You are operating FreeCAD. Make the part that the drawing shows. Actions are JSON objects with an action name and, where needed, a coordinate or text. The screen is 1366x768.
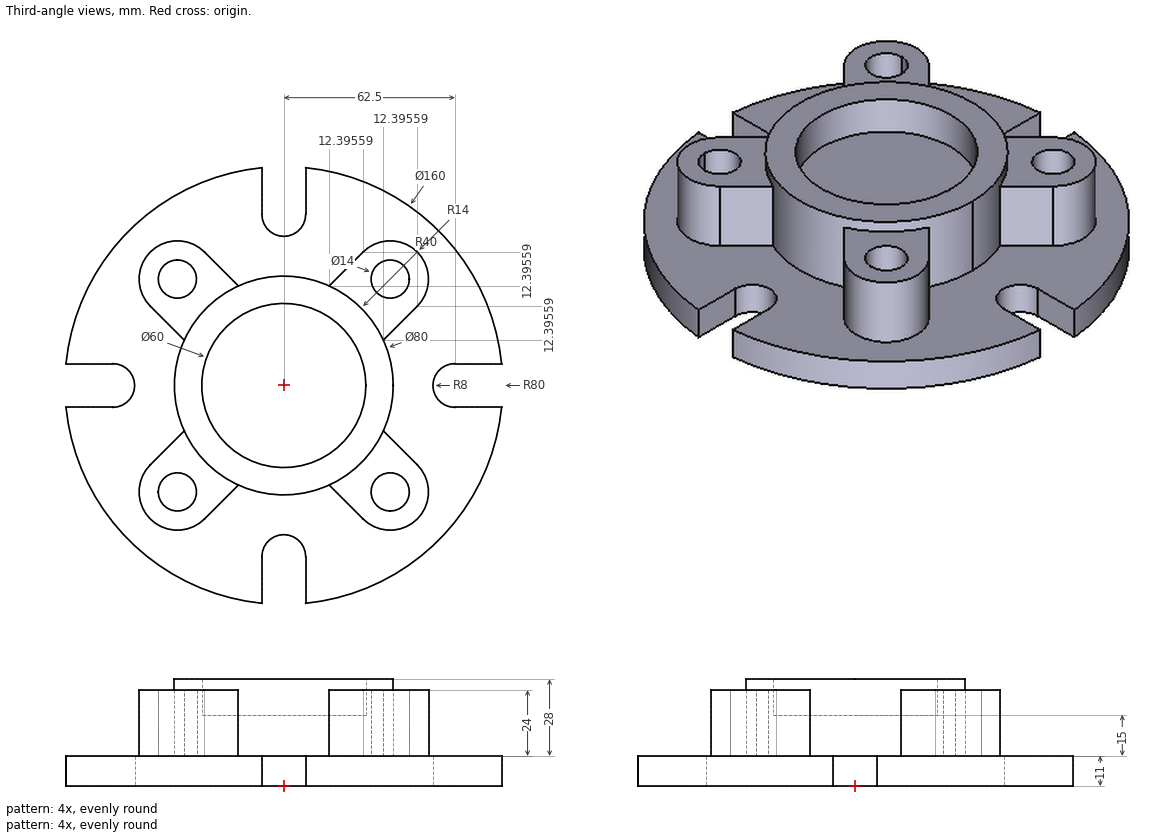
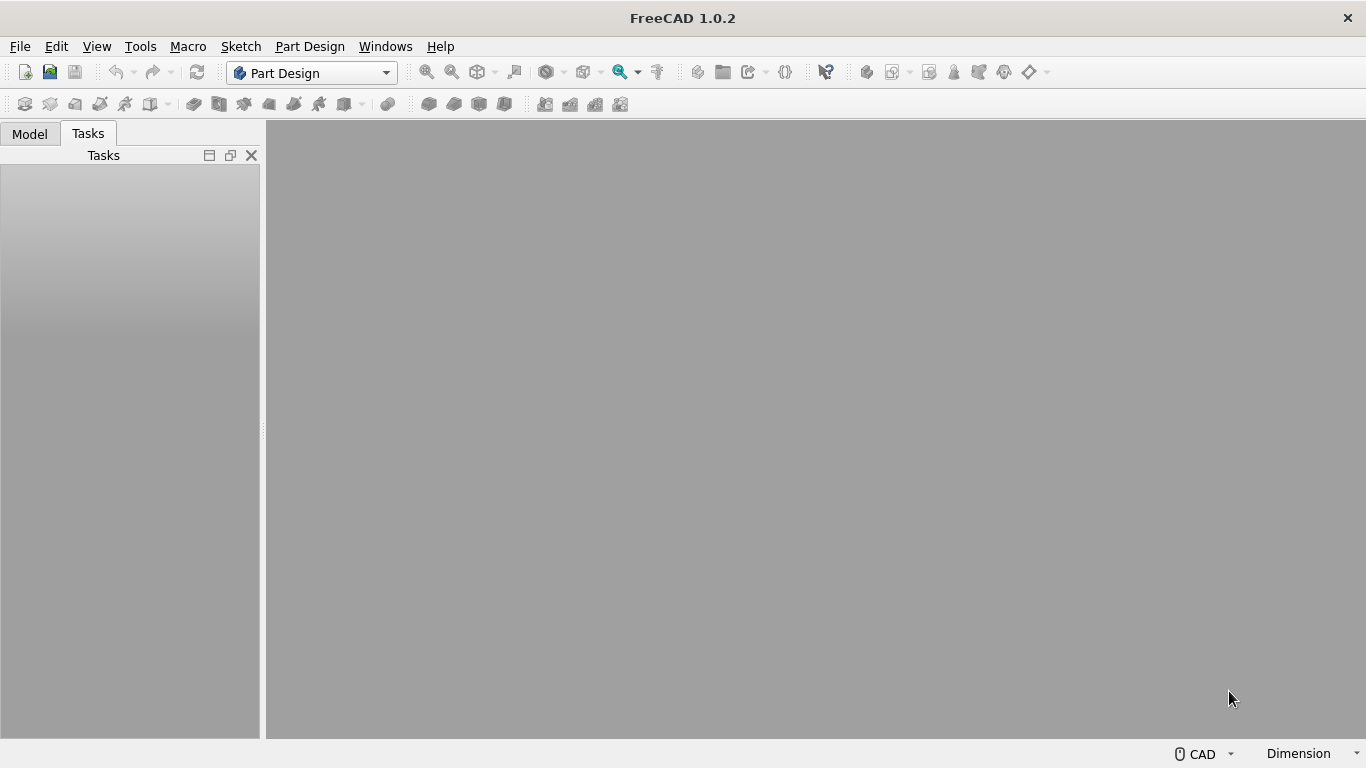
{"action": "left_click", "coordinate": [25, 72]}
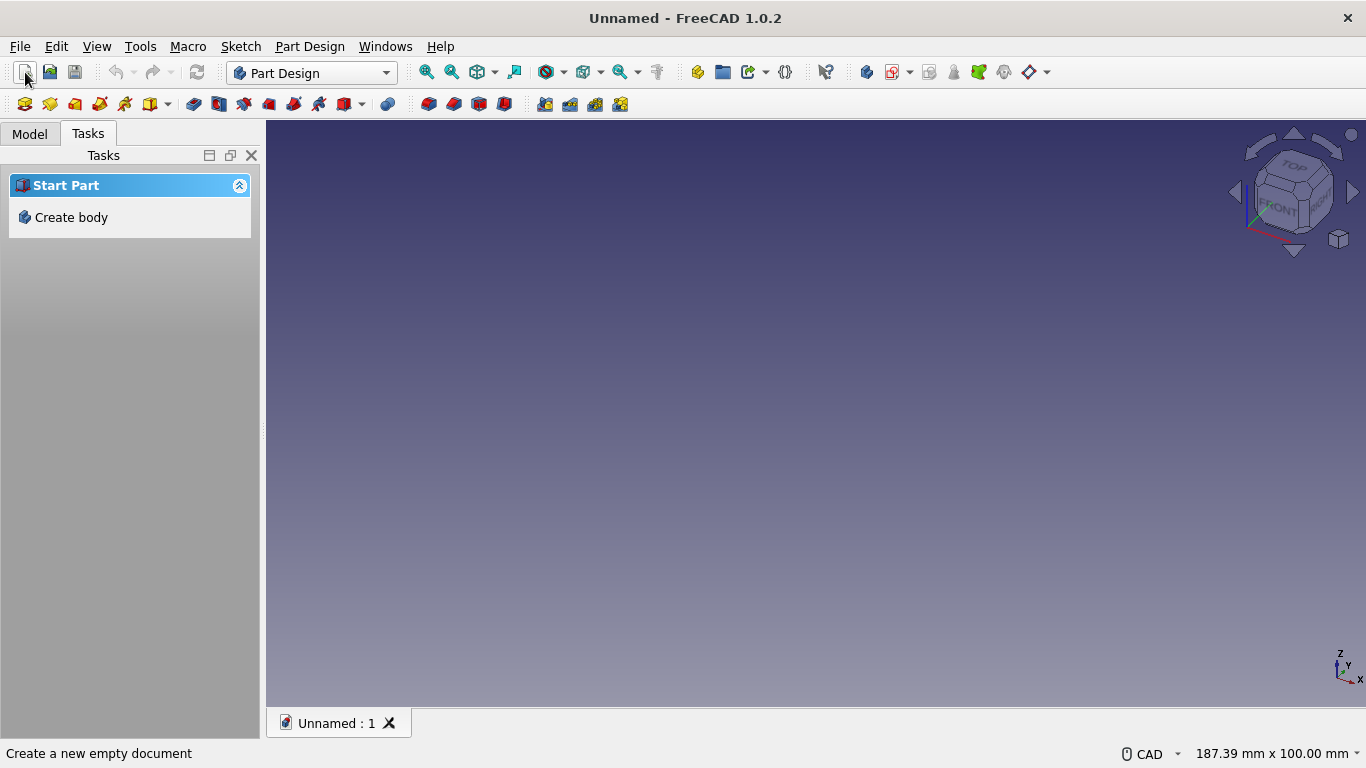
{"action": "left_click", "coordinate": [892, 72]}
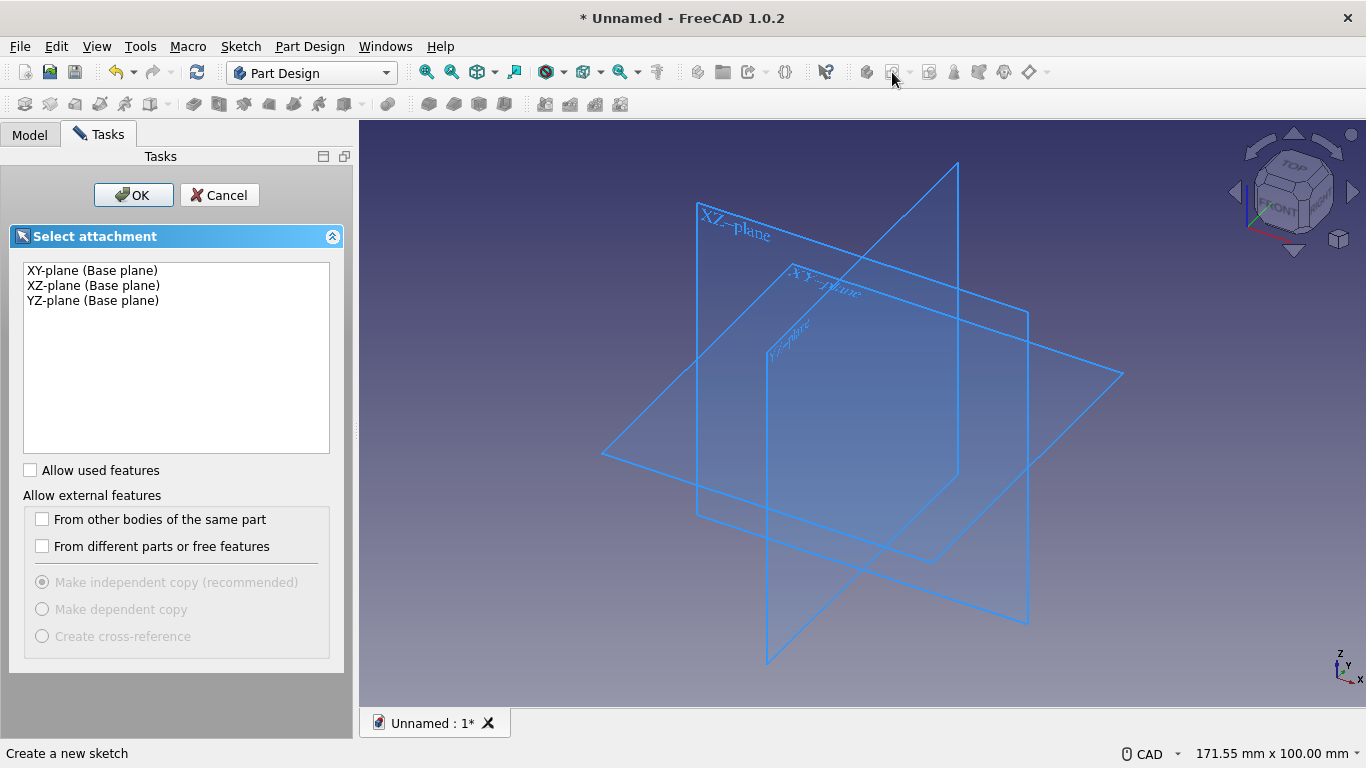
{"action": "left_click", "coordinate": [84, 270]}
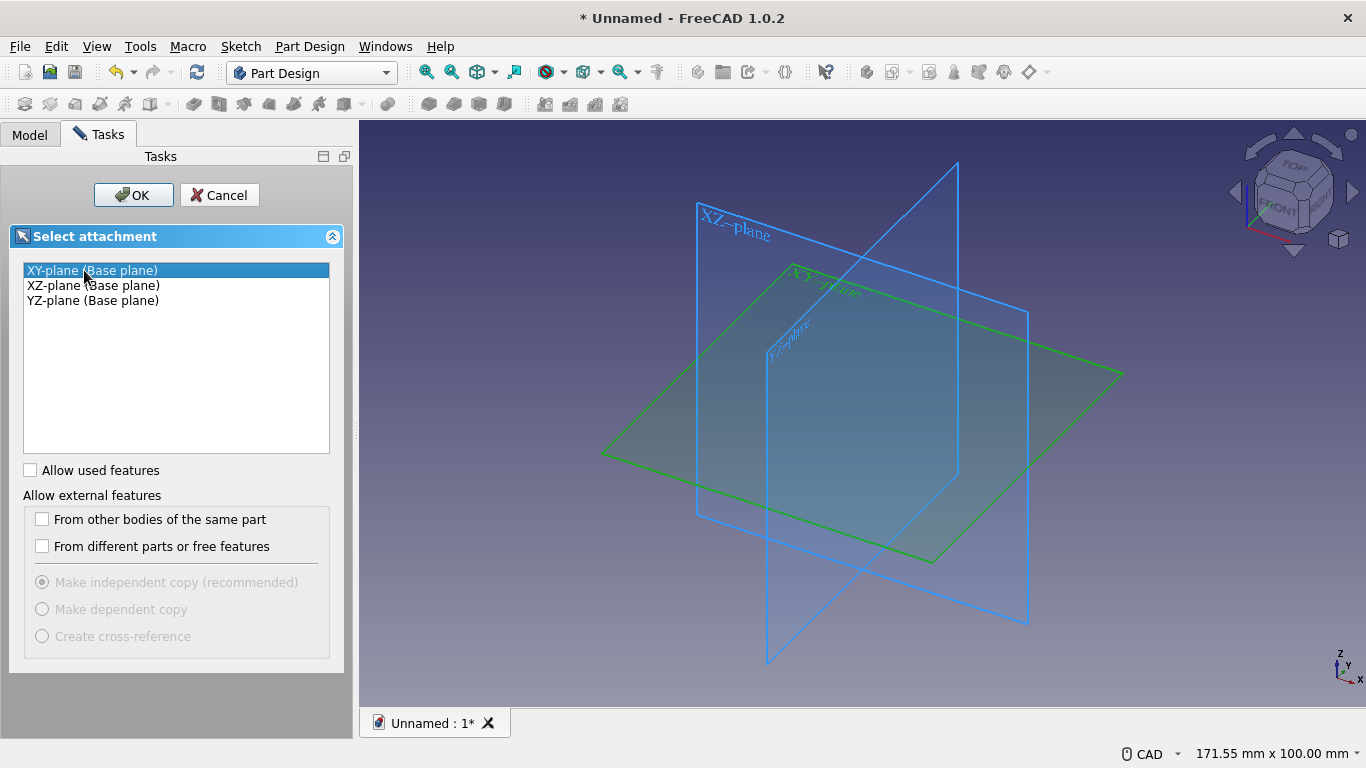
{"action": "left_click", "coordinate": [134, 195]}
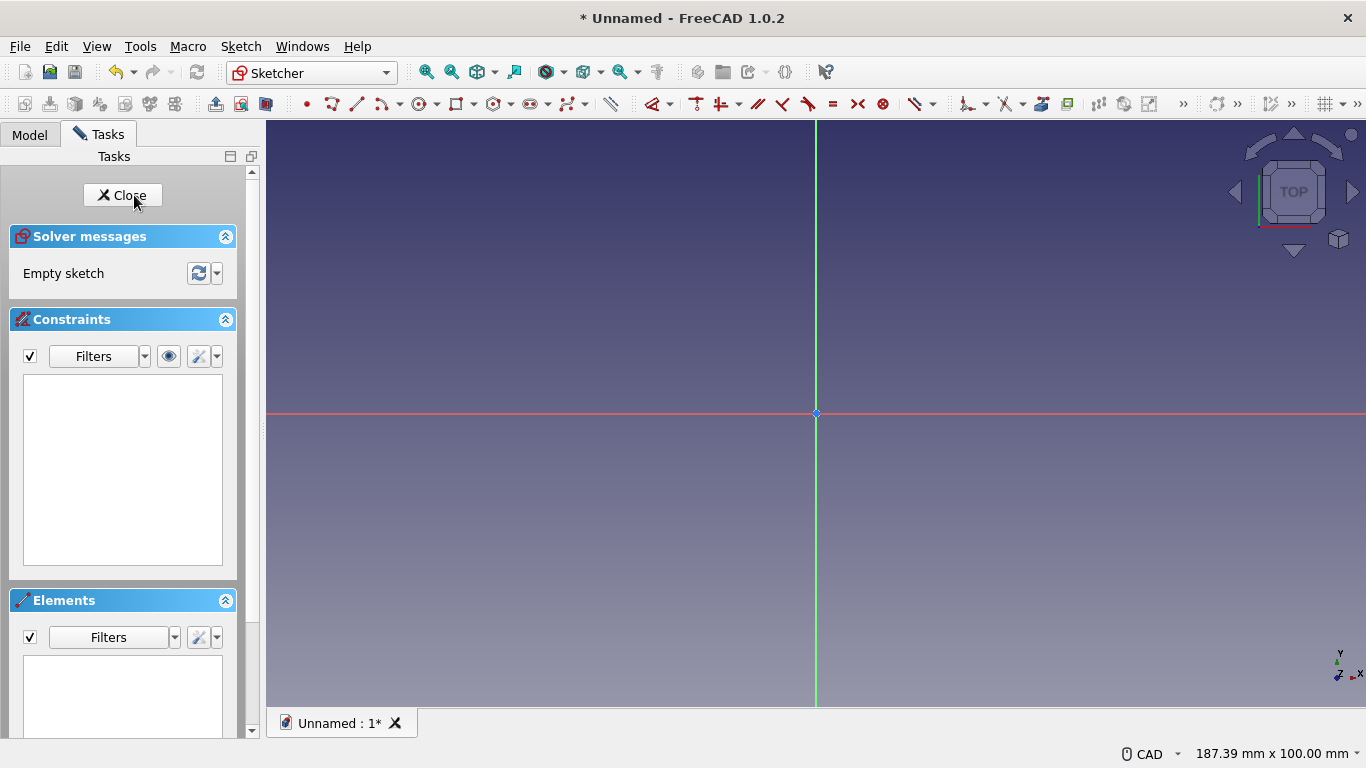
{"action": "scroll", "coordinate": [708, 414], "scroll_direction": "down", "scroll_amount": 5}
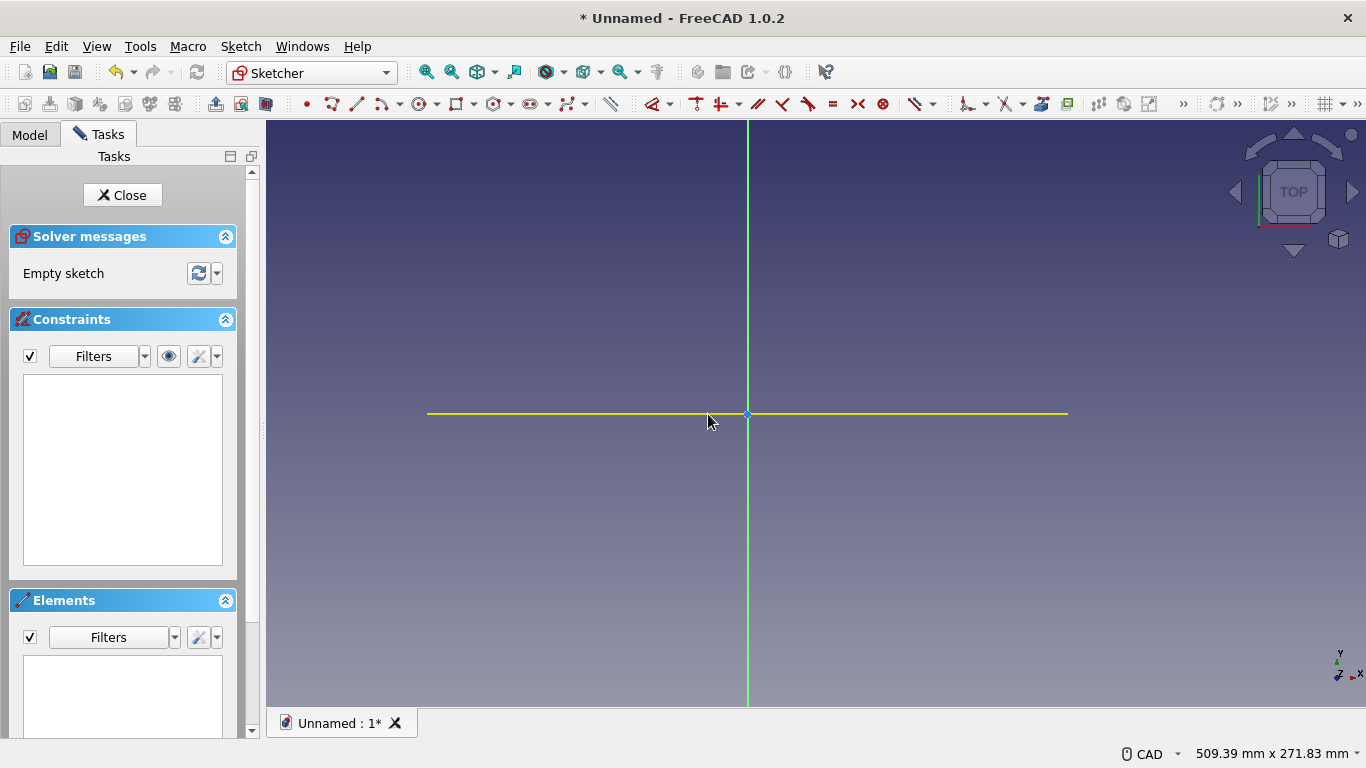
{"action": "key", "text": "g c"}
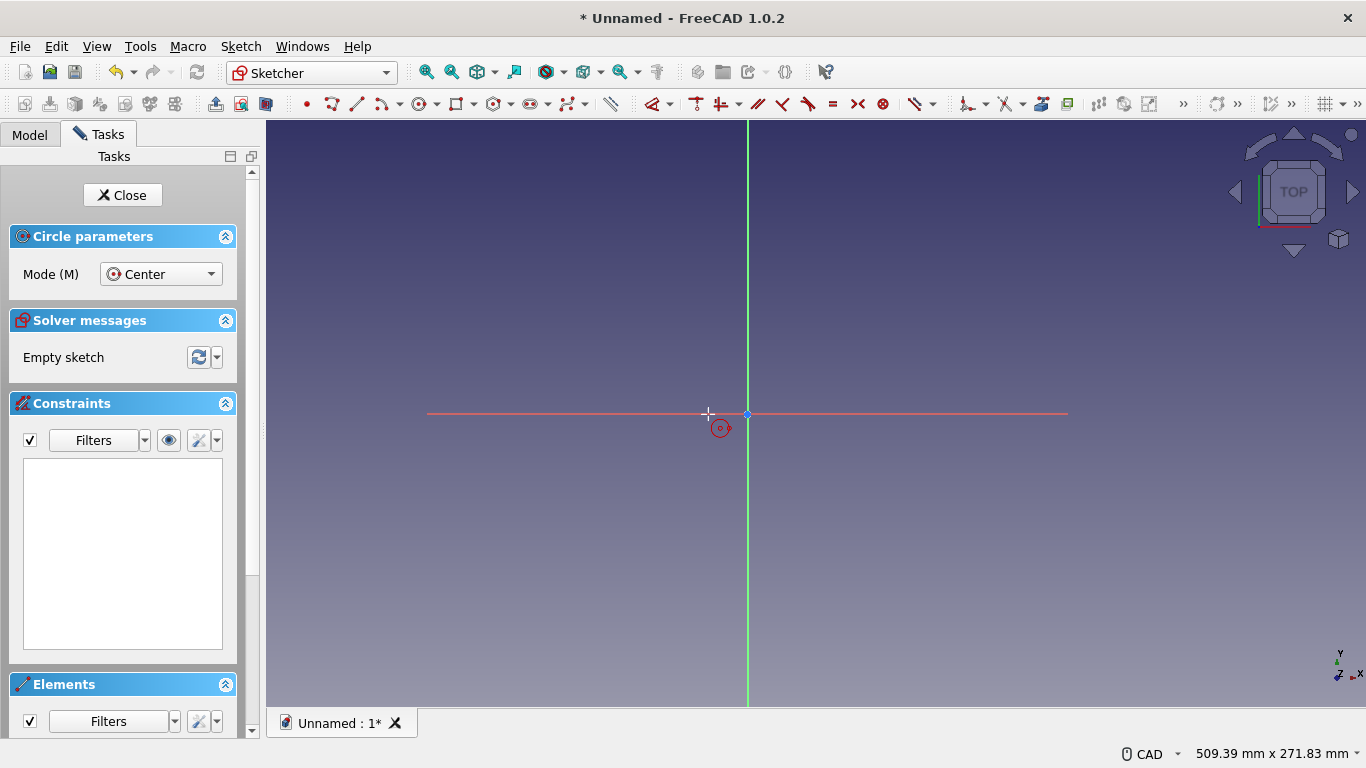
{"action": "left_click", "coordinate": [748, 414]}
{"action": "left_click", "coordinate": [870, 292]}
{"action": "key", "text": "Escape"}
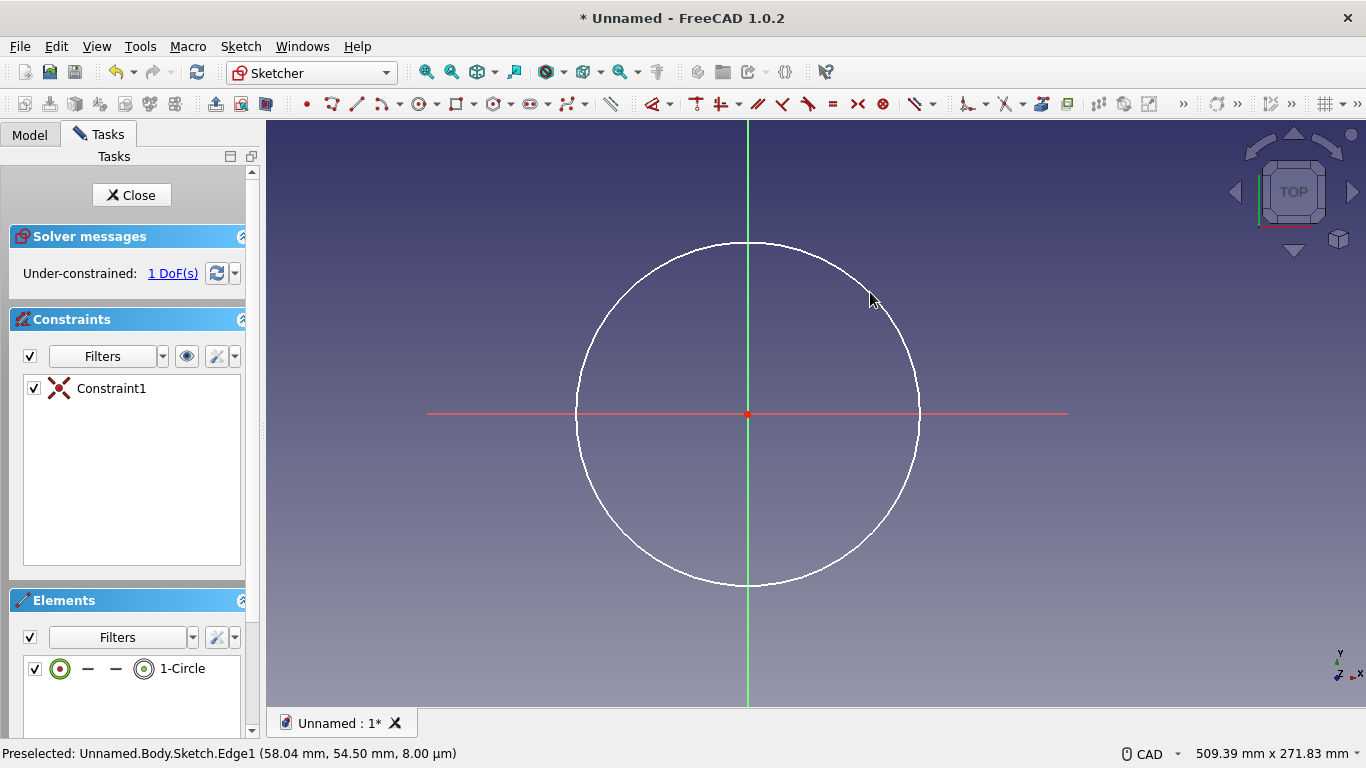
{"action": "key", "text": "d"}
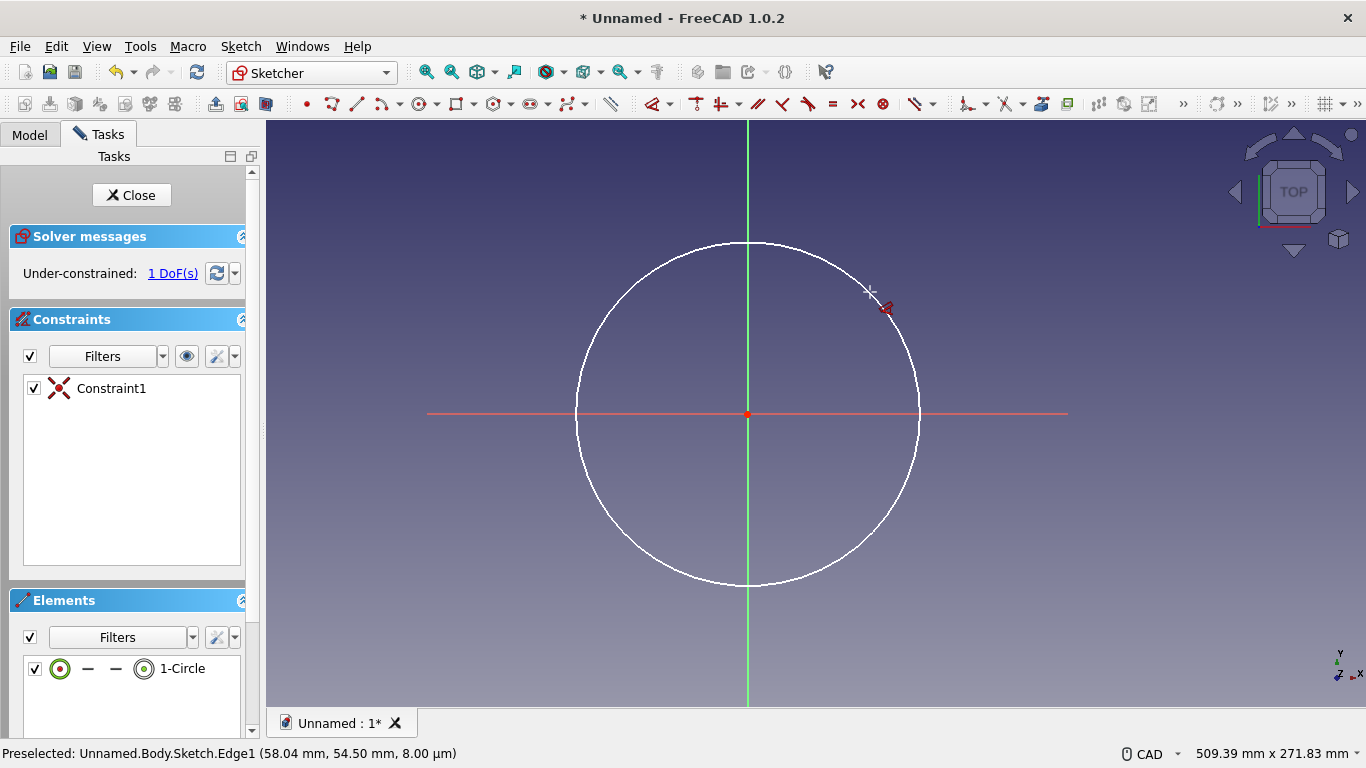
{"action": "left_click", "coordinate": [869, 292]}
{"action": "left_click", "coordinate": [892, 269]}